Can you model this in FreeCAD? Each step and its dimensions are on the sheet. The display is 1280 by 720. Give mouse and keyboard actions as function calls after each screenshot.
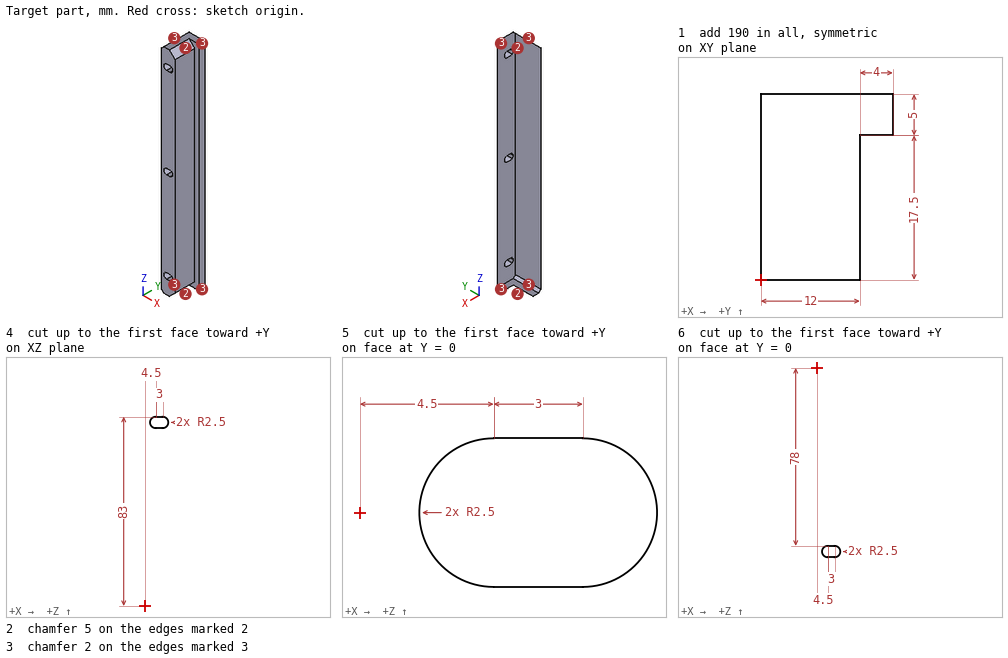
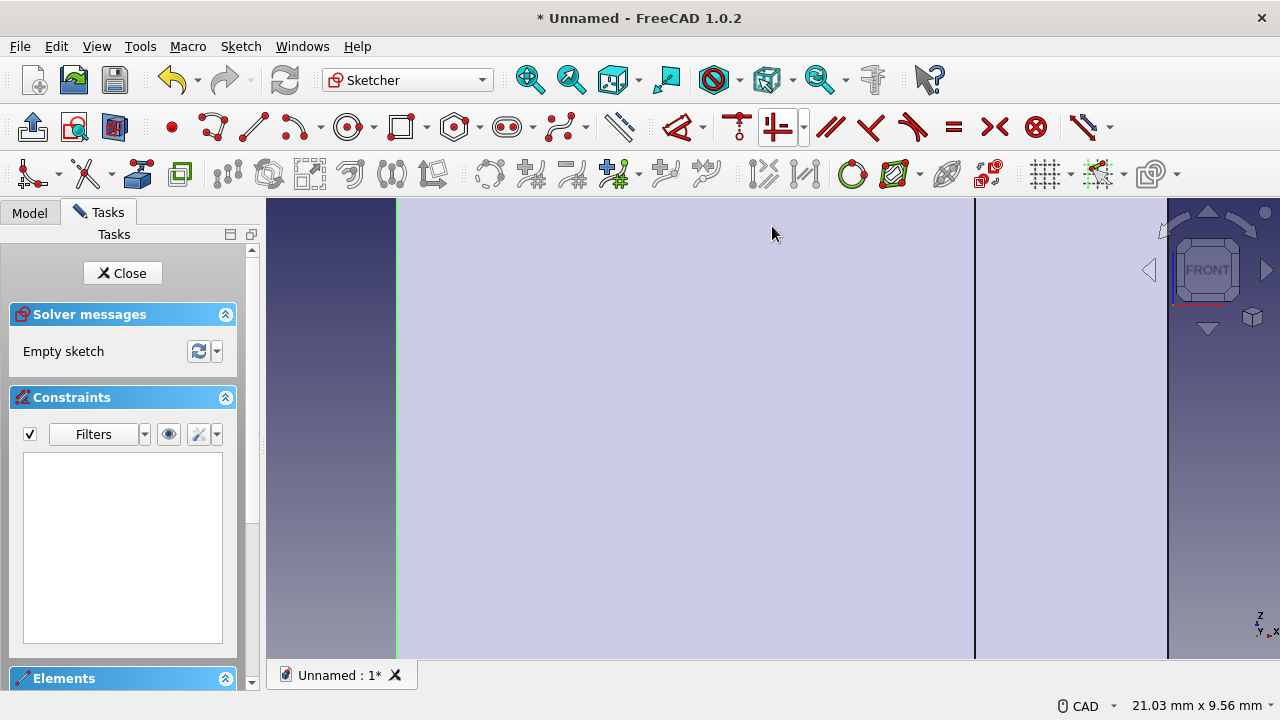
click(506, 128)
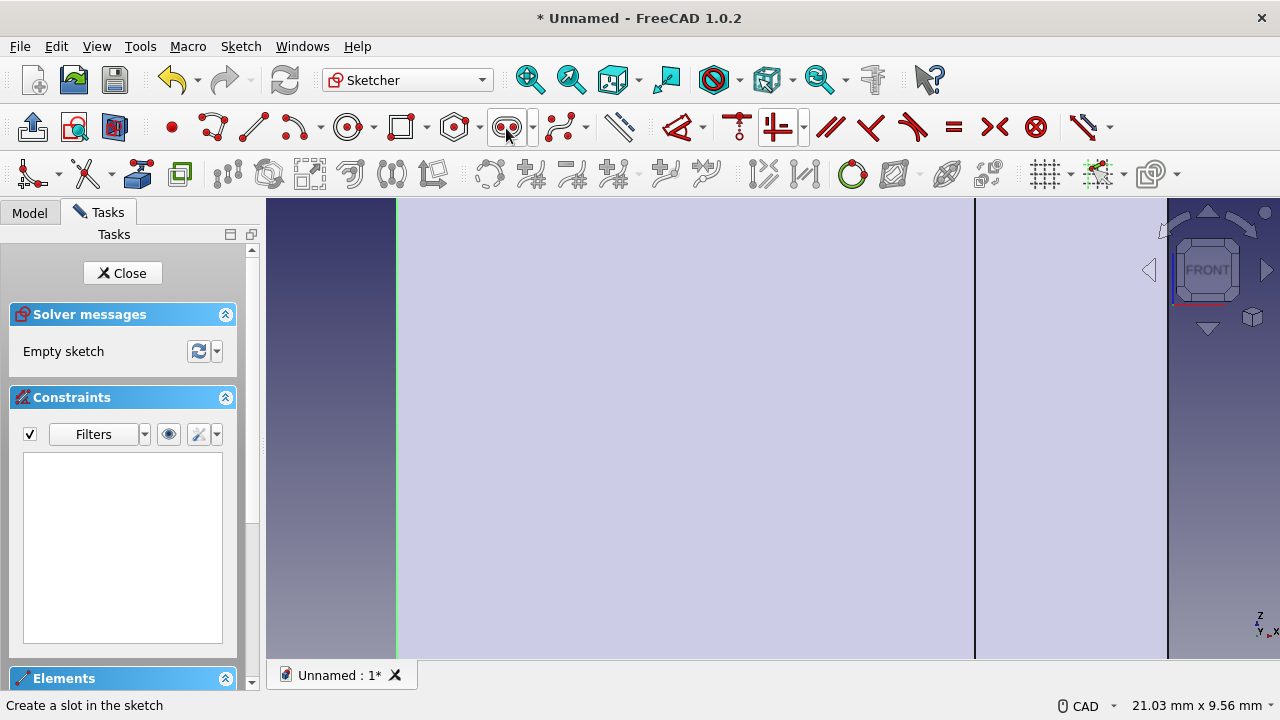
click(614, 410)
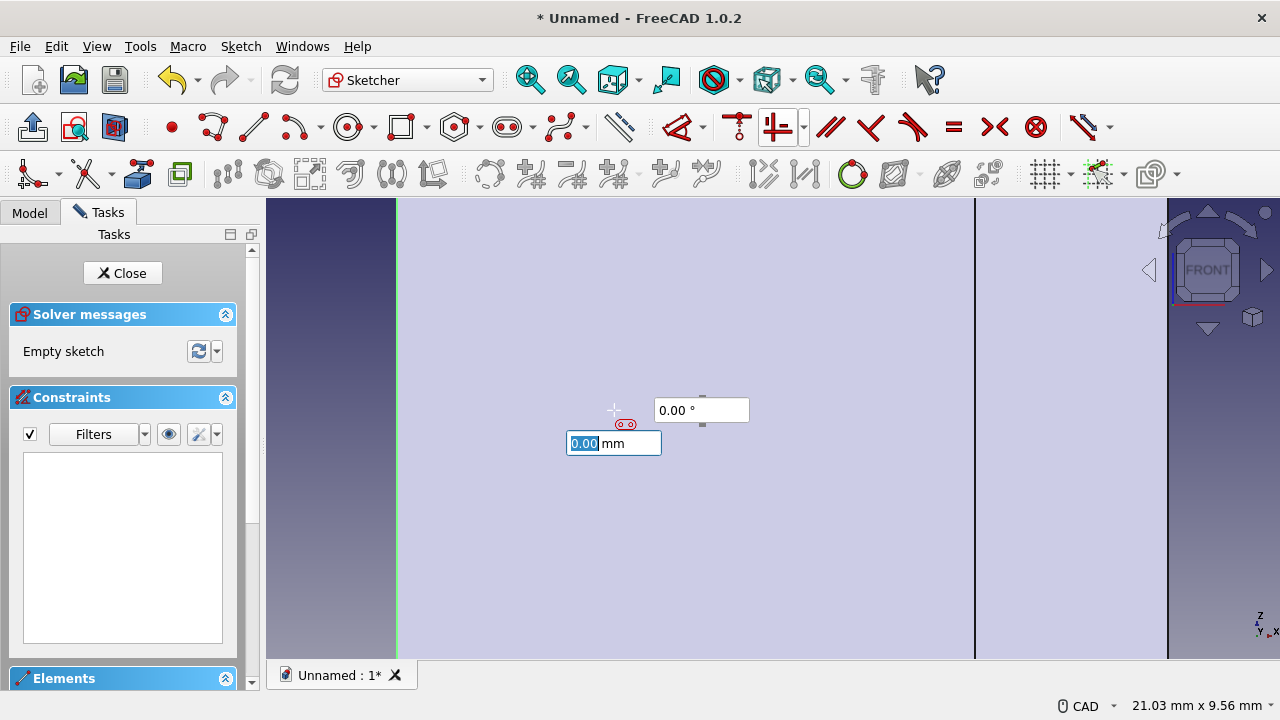
click(758, 410)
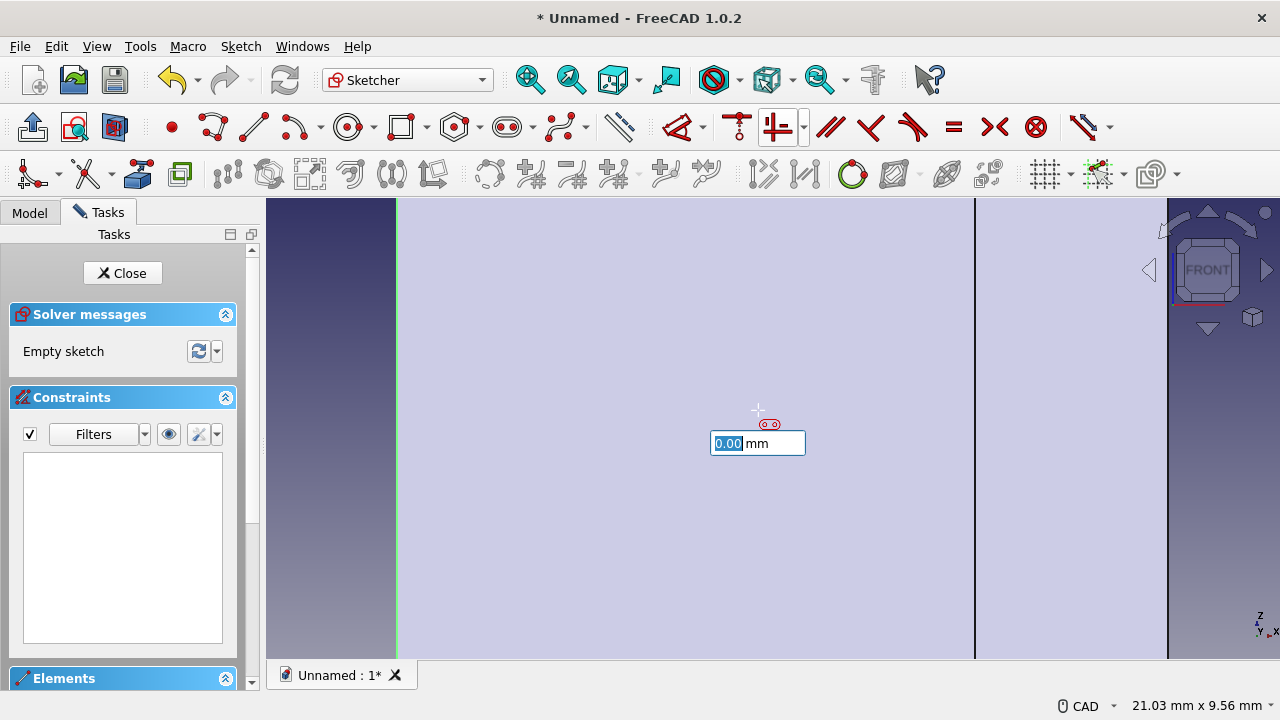
click(686, 289)
key(Escape)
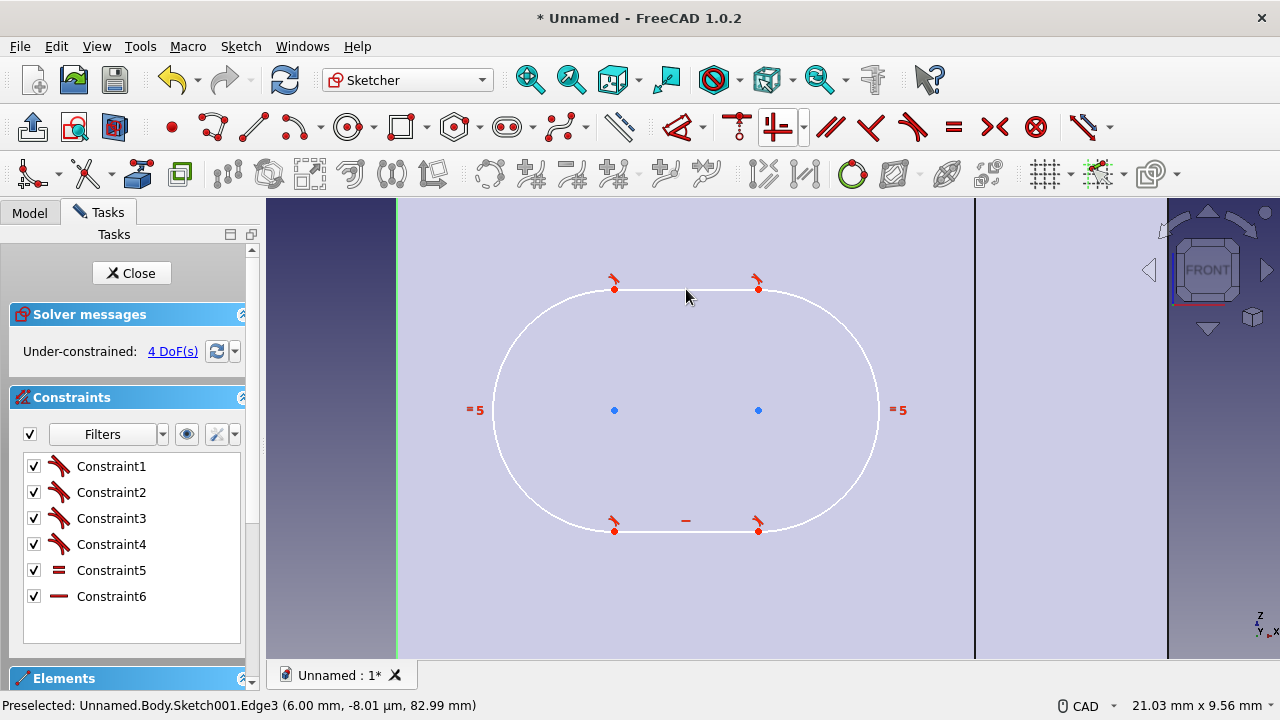
click(676, 128)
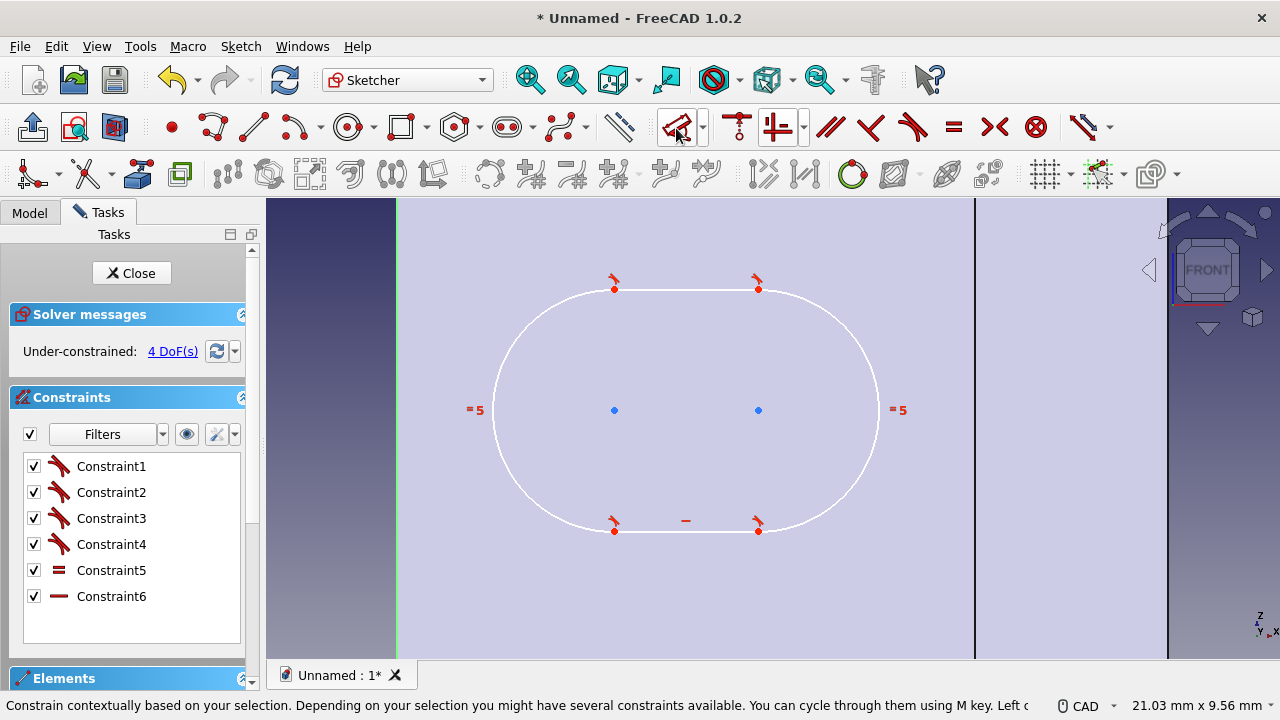
click(516, 340)
click(490, 321)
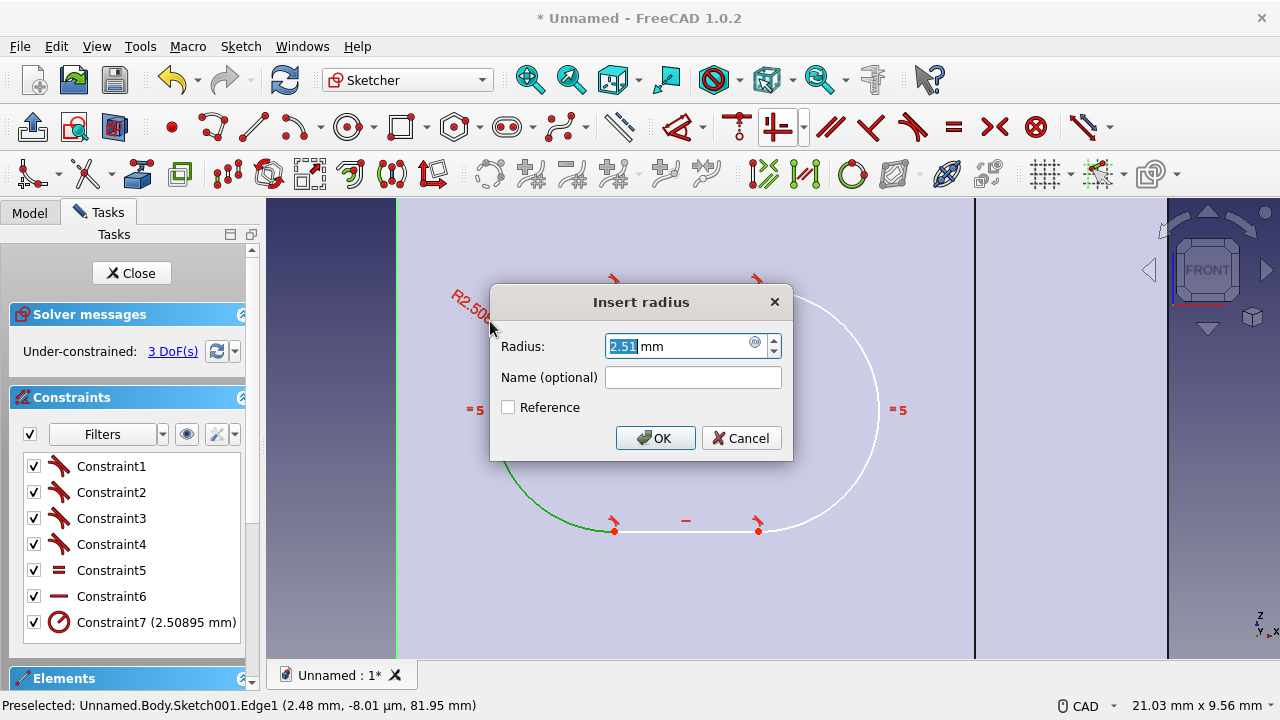
text(2.5)
key(Return)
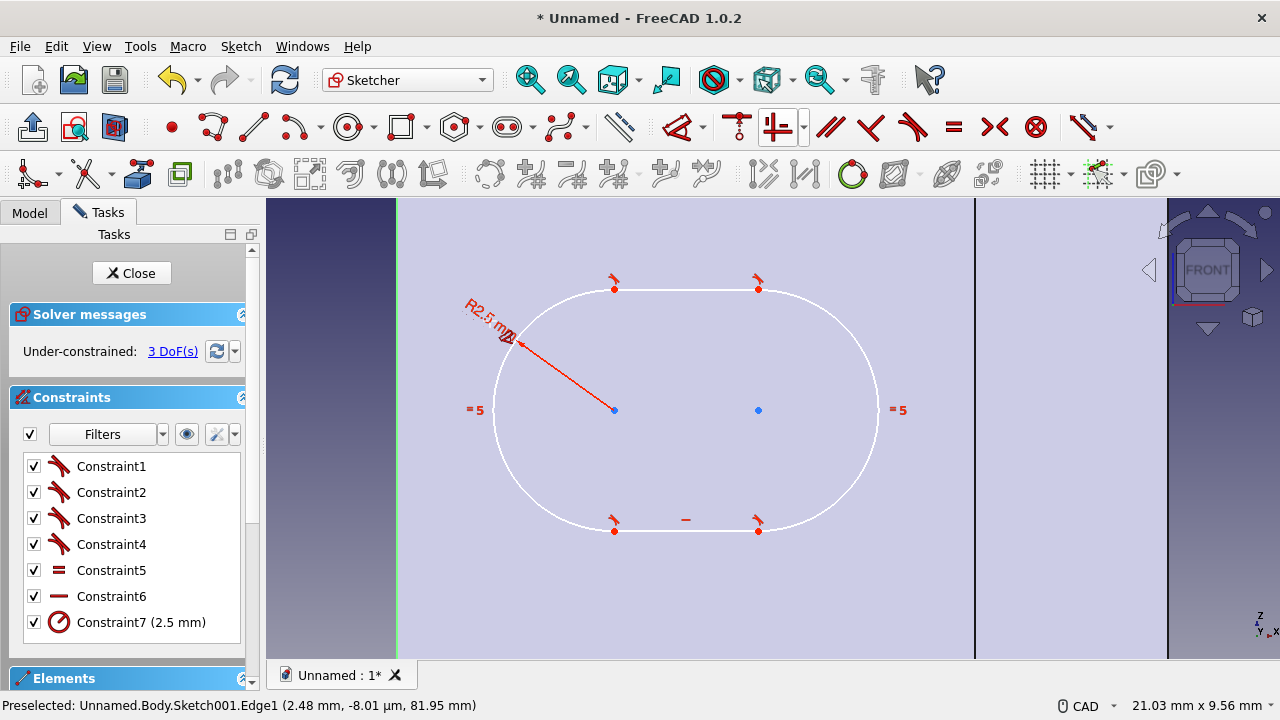
click(657, 290)
click(686, 256)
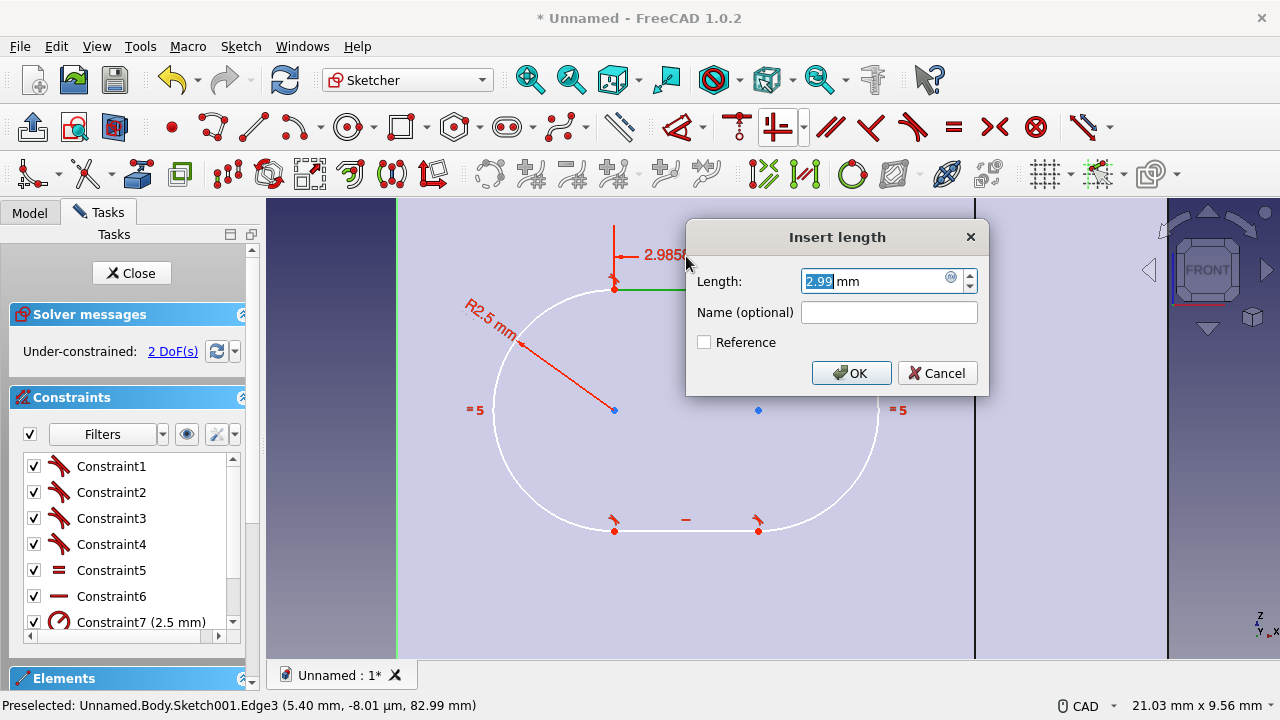
text(3)
key(Return)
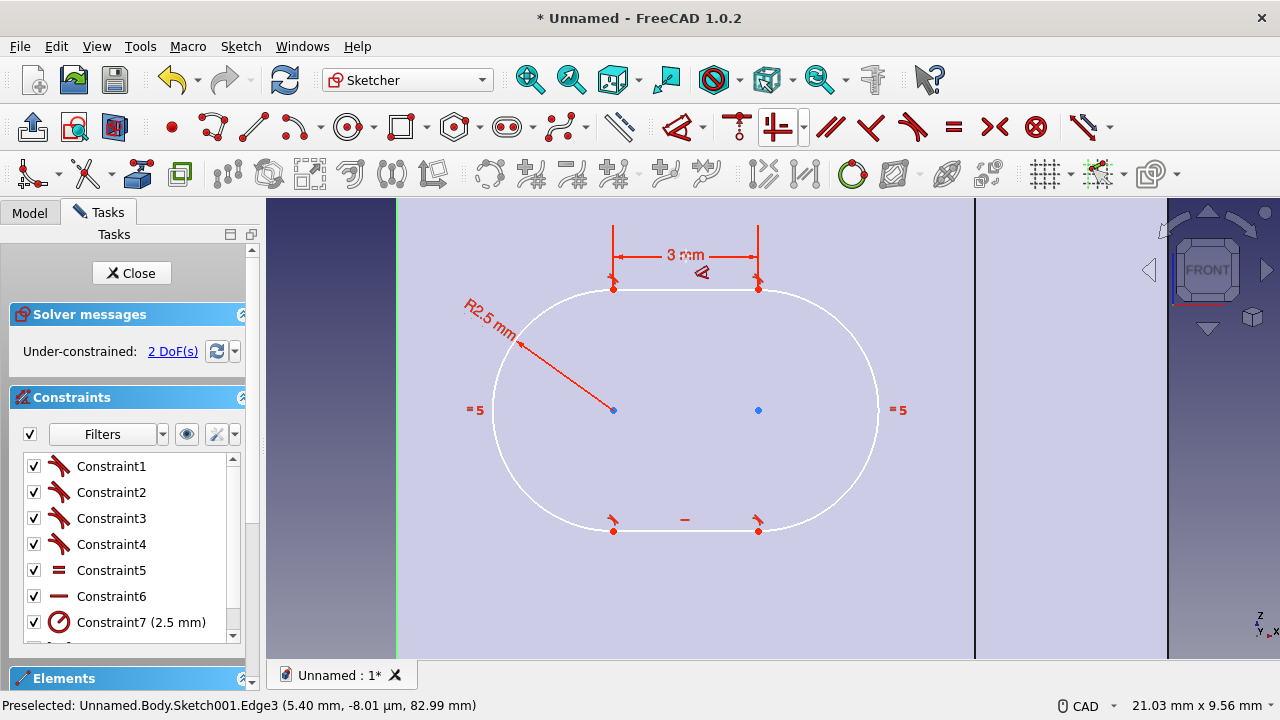
click(613, 290)
click(363, 461)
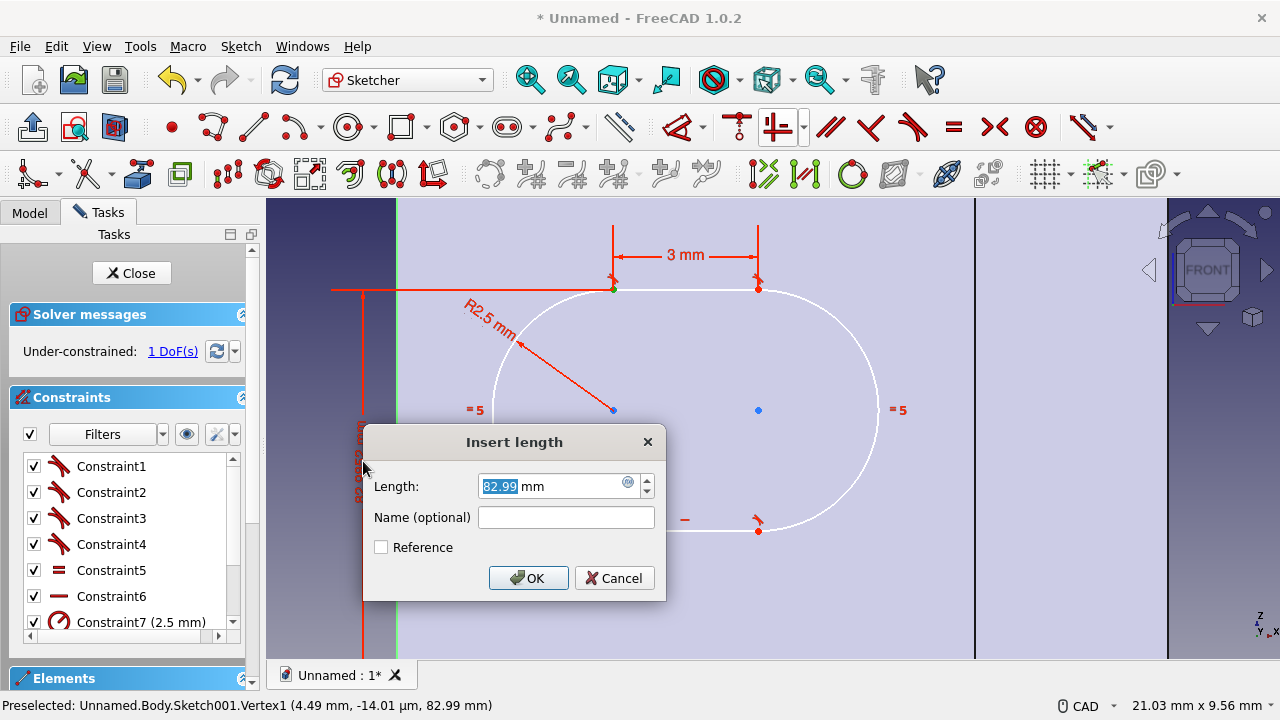
text(83)
key(Return)